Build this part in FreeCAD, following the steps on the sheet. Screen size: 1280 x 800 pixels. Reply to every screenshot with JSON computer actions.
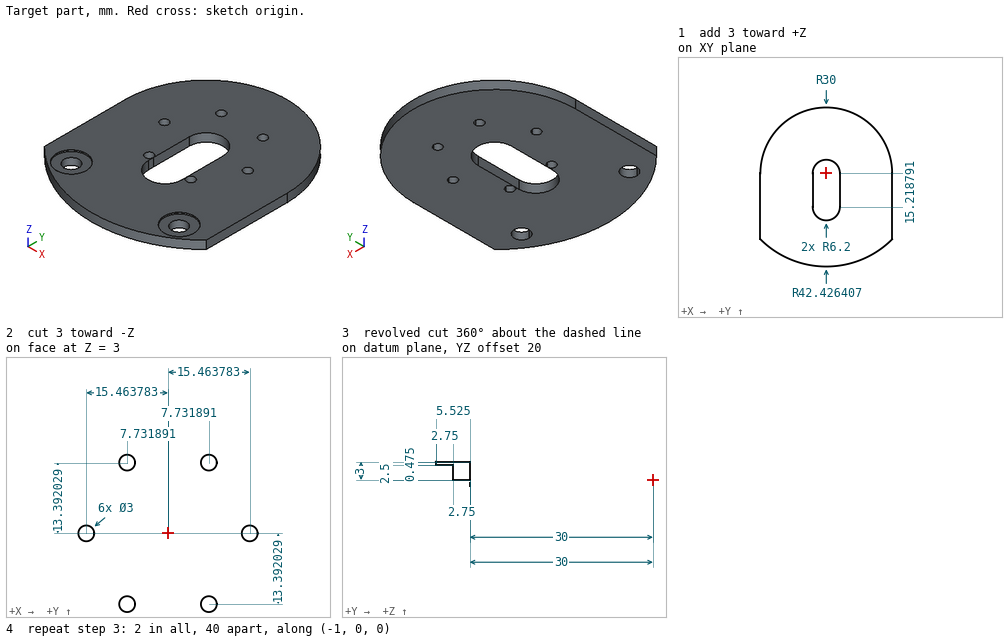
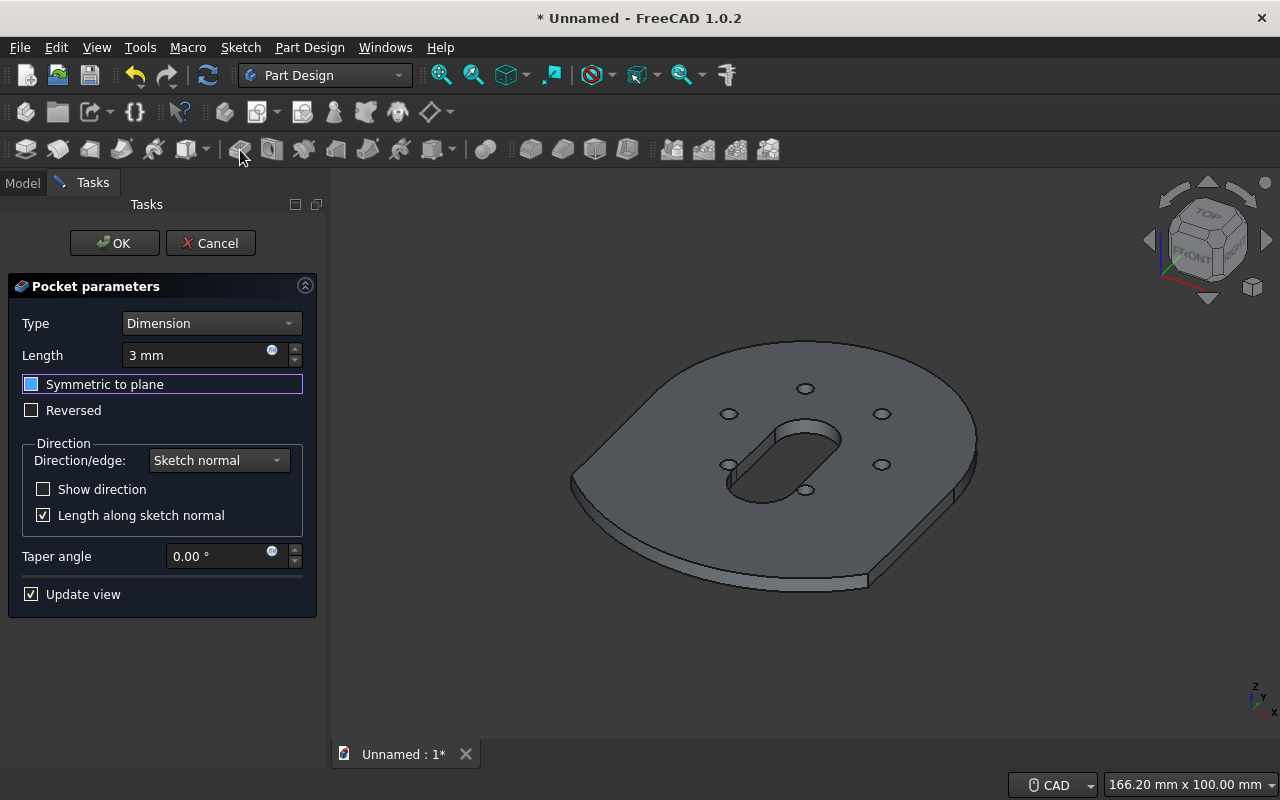
{"action": "left_click", "coordinate": [115, 243]}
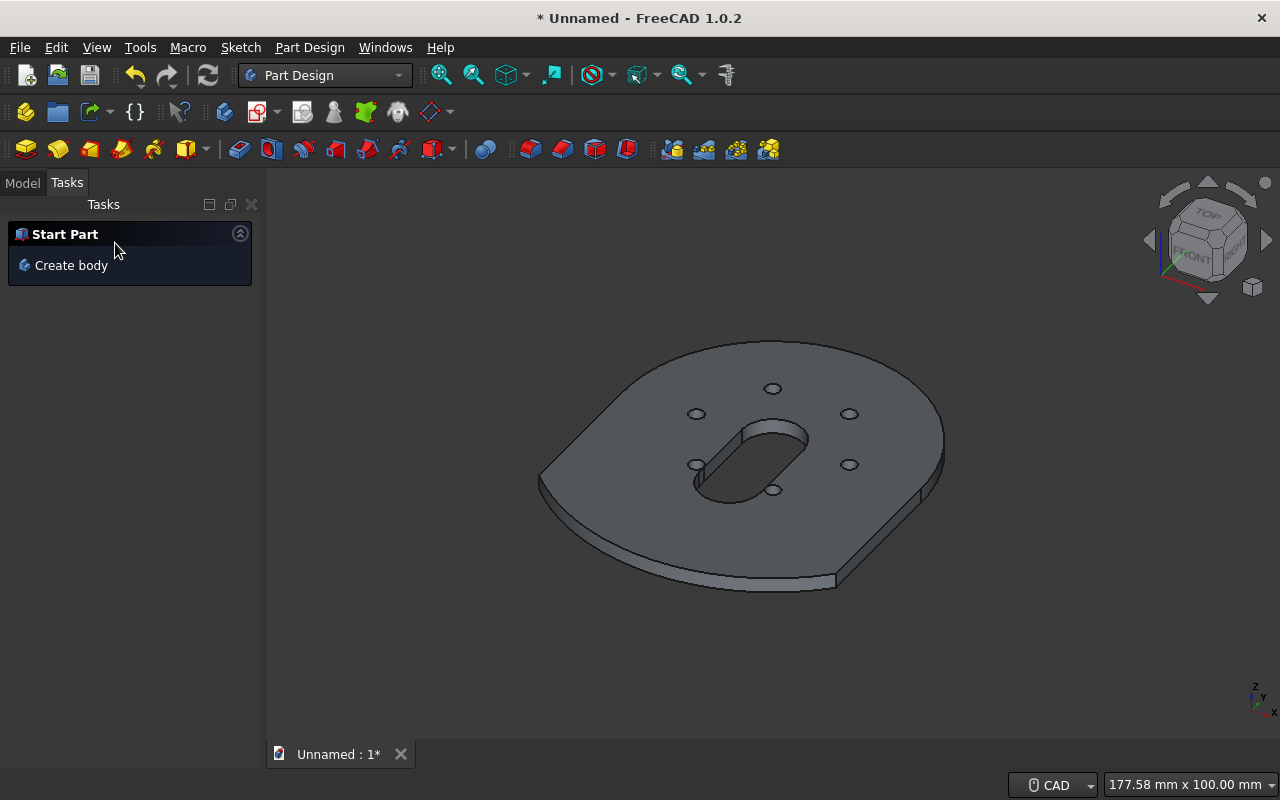
{"action": "left_click", "coordinate": [23, 182]}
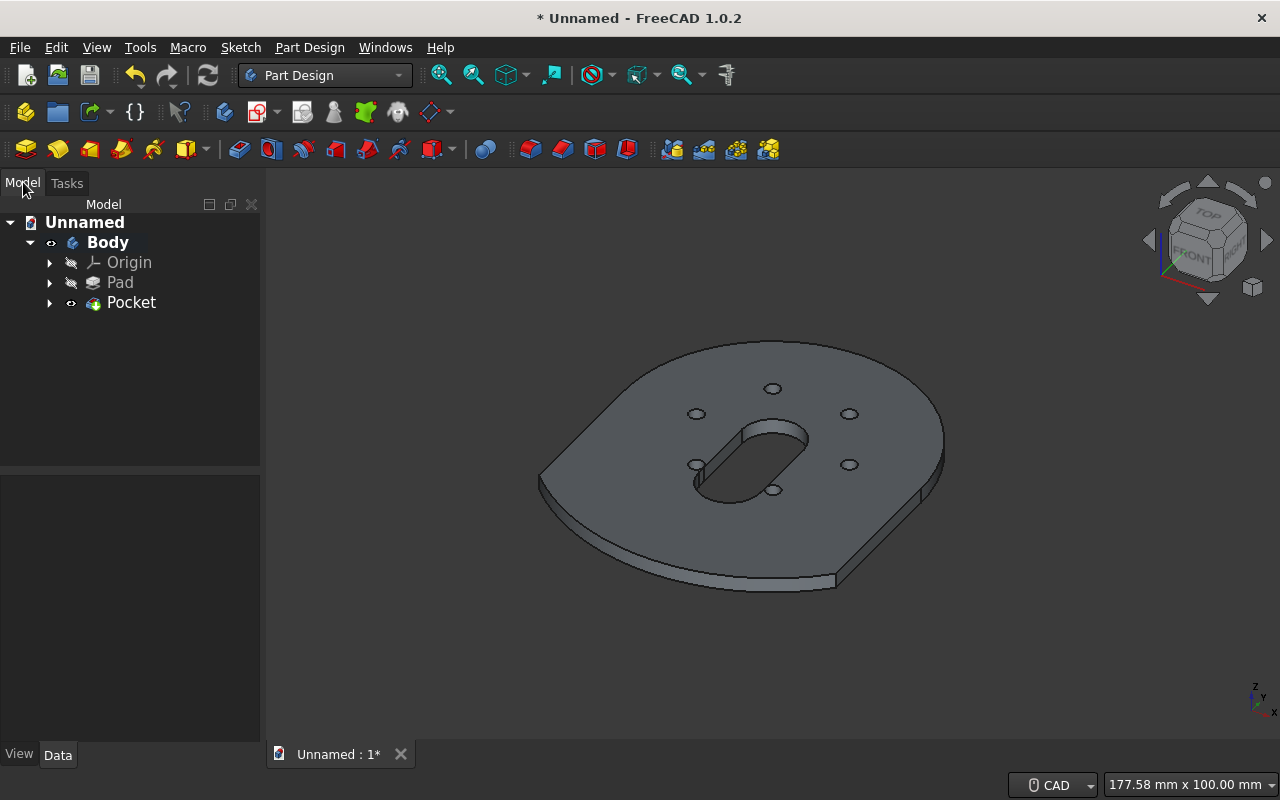
{"action": "left_click", "coordinate": [50, 263]}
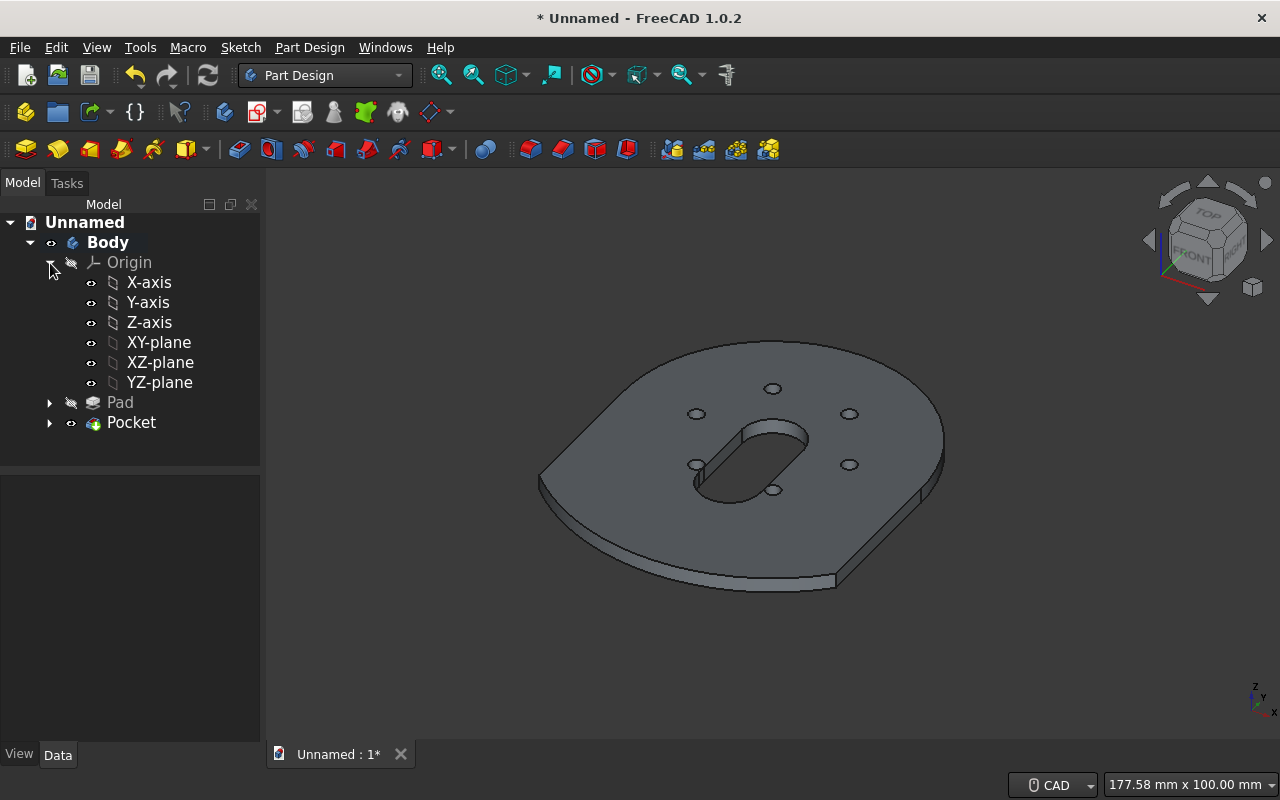
{"action": "left_click", "coordinate": [136, 383]}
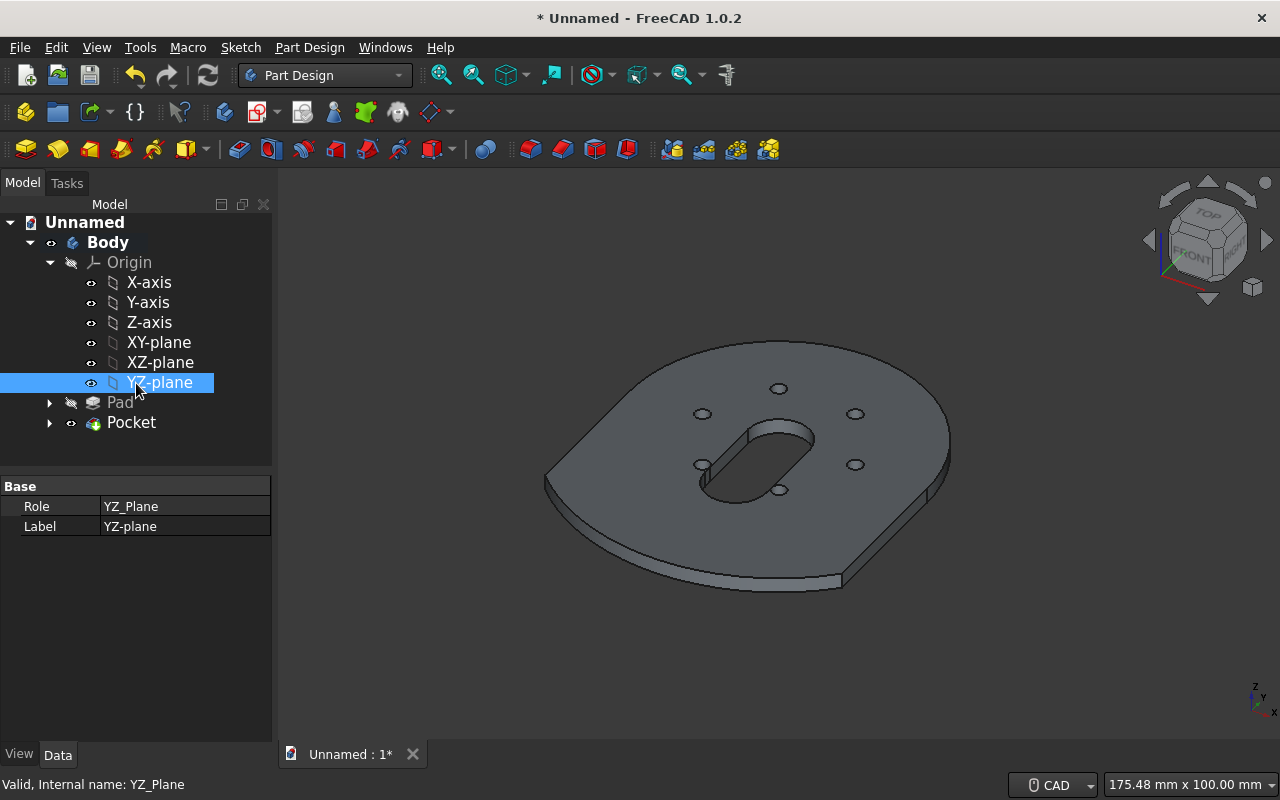
{"action": "left_click", "coordinate": [430, 112]}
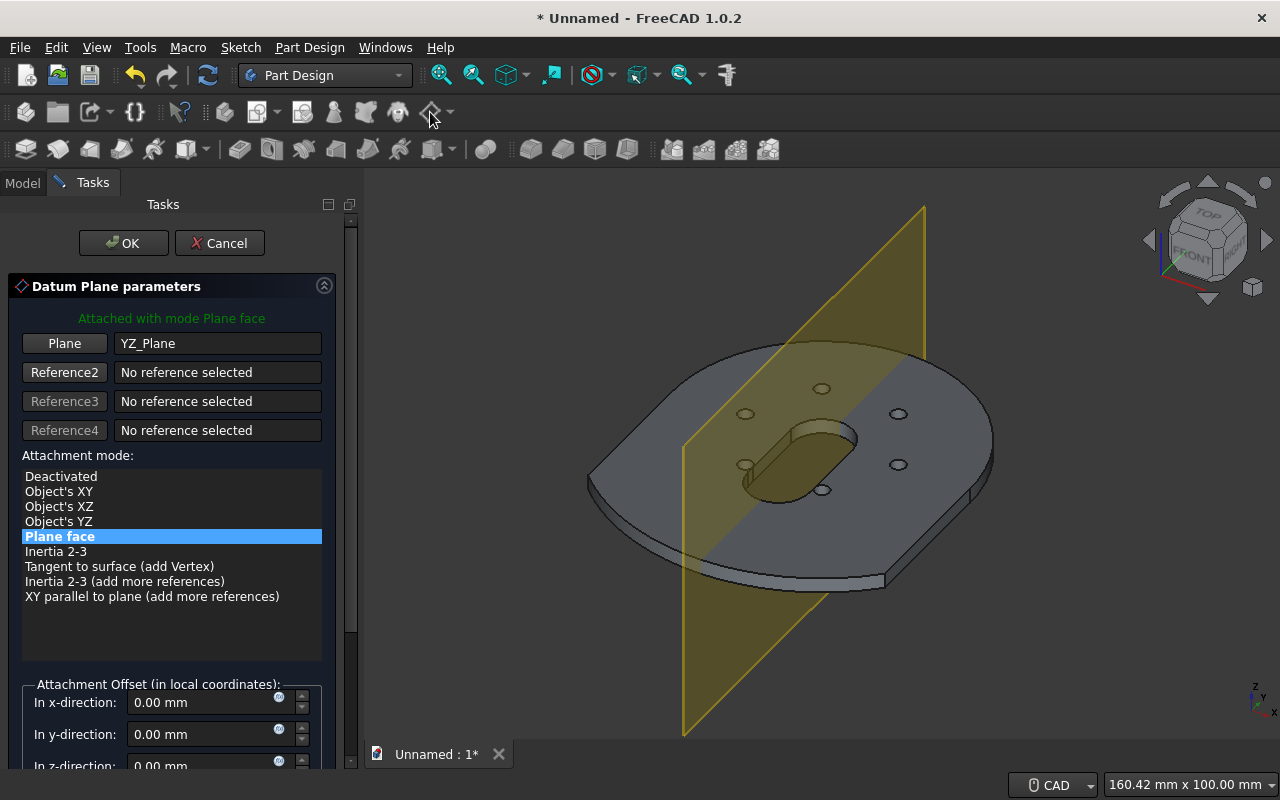
{"action": "scroll", "coordinate": [351, 491], "scroll_direction": "down", "scroll_amount": 2}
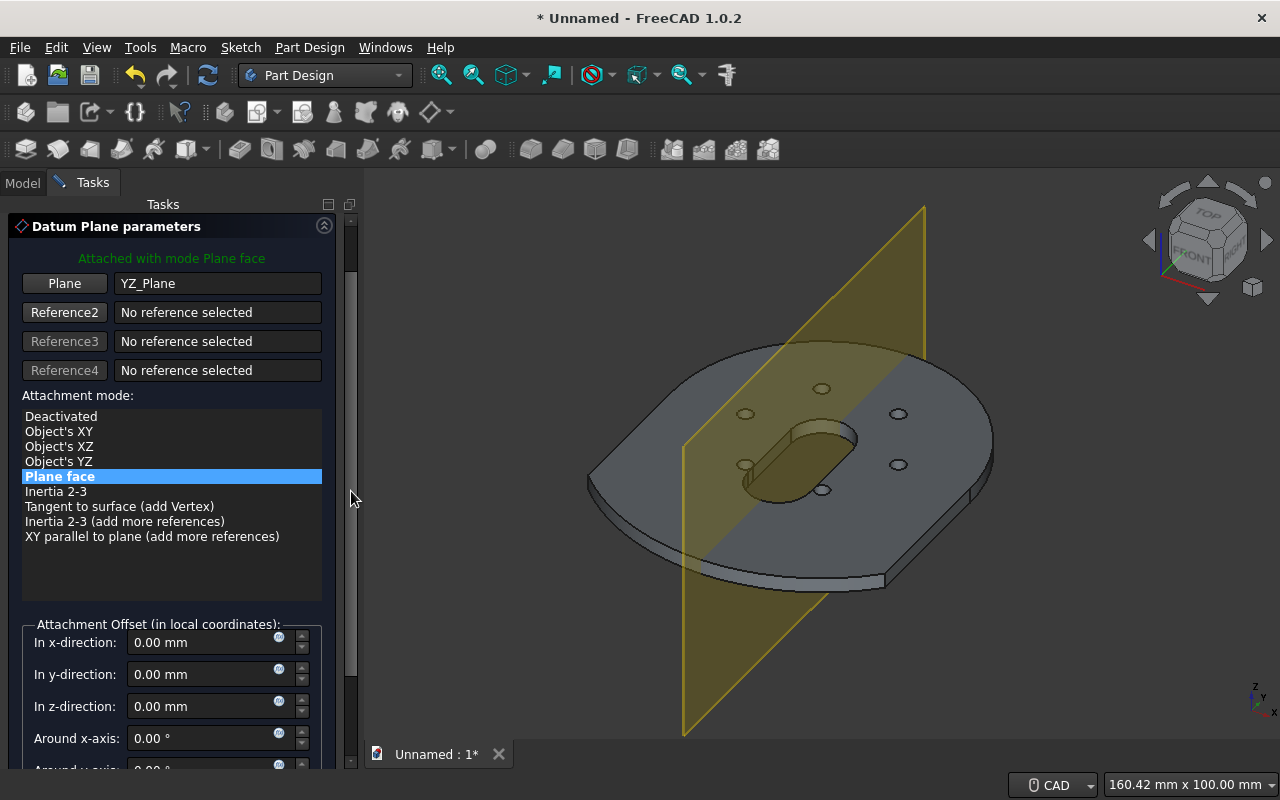
{"action": "triple_click", "coordinate": [210, 646]}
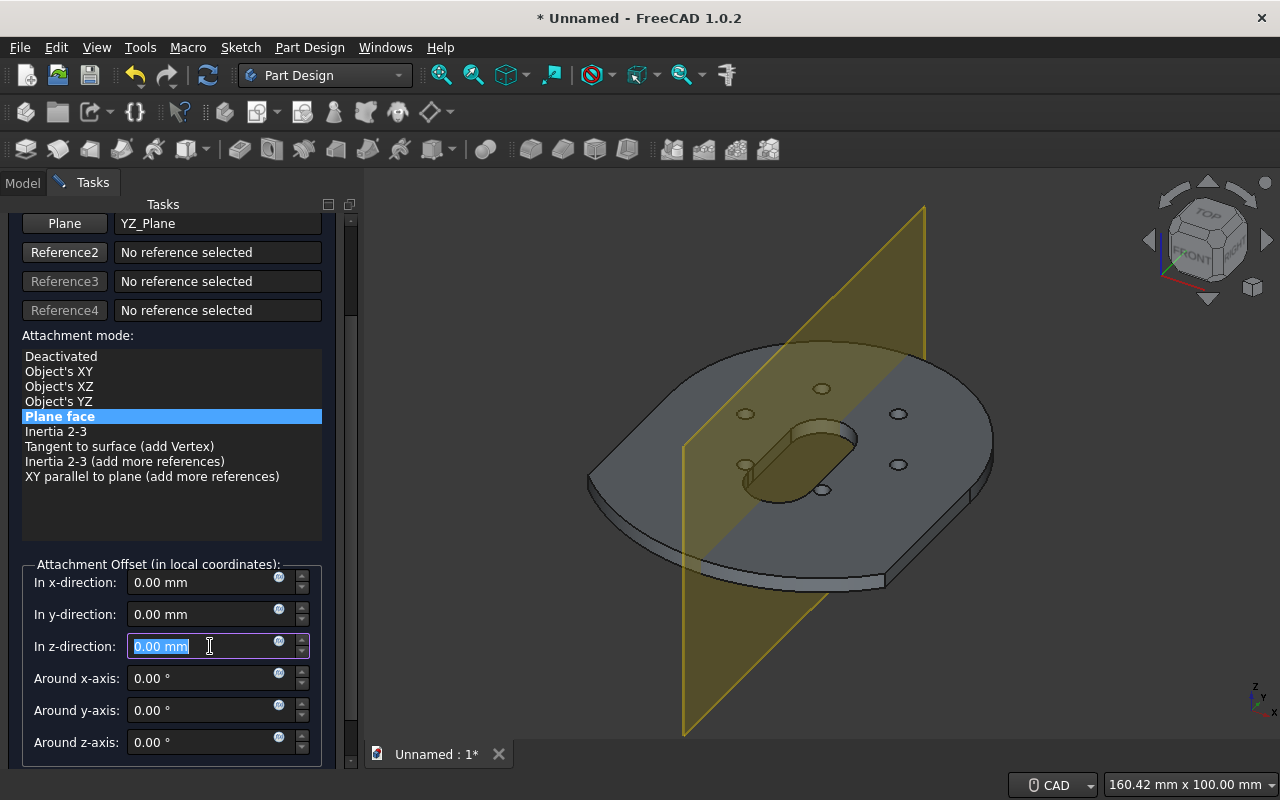
{"action": "type", "text": "20"}
{"action": "key", "text": "Tab"}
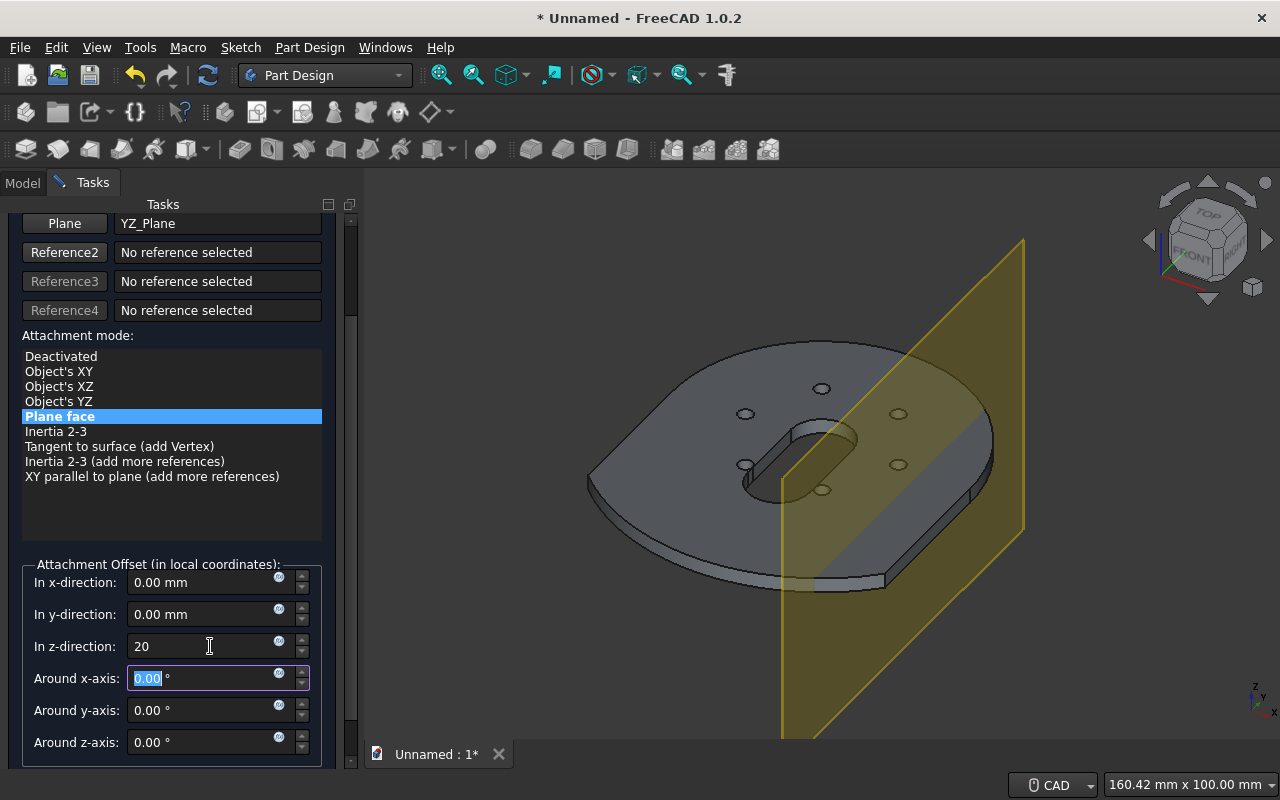
{"action": "scroll", "coordinate": [351, 491], "scroll_direction": "up", "scroll_amount": 3}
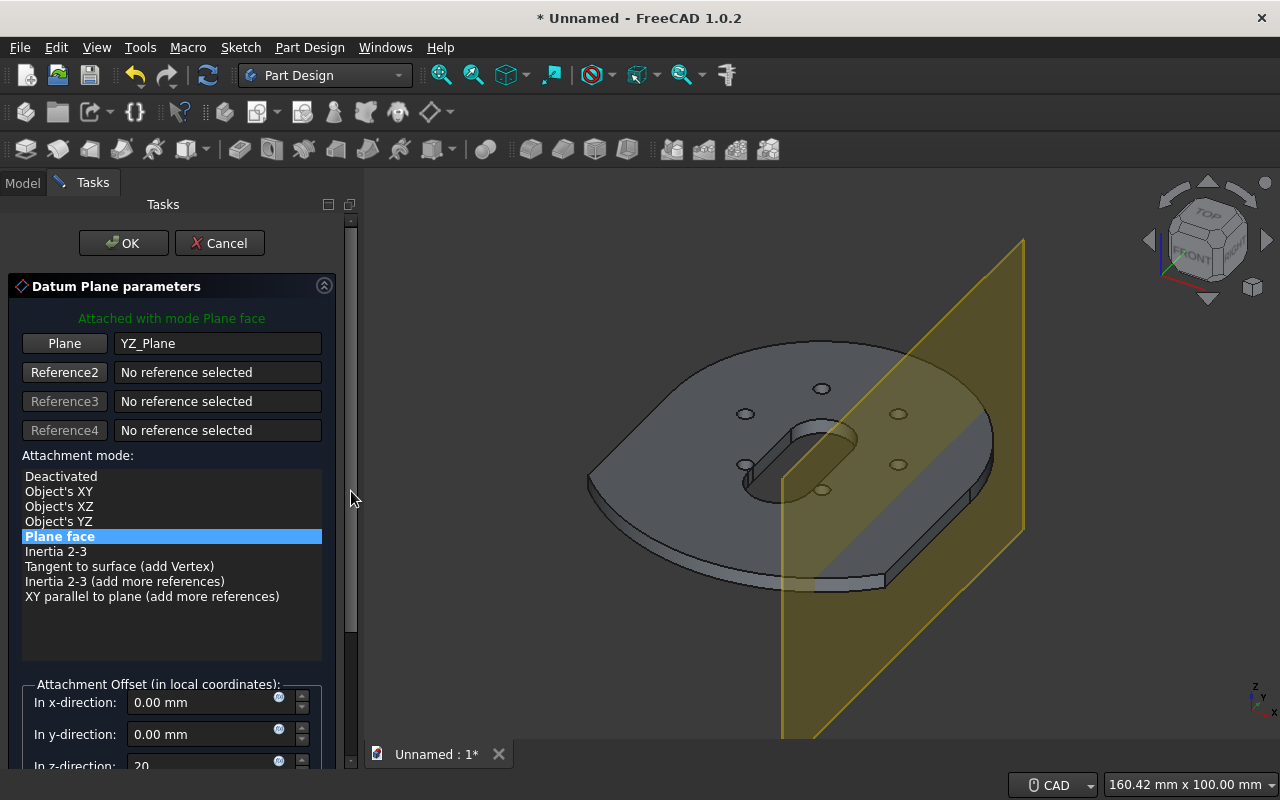
{"action": "left_click", "coordinate": [124, 243]}